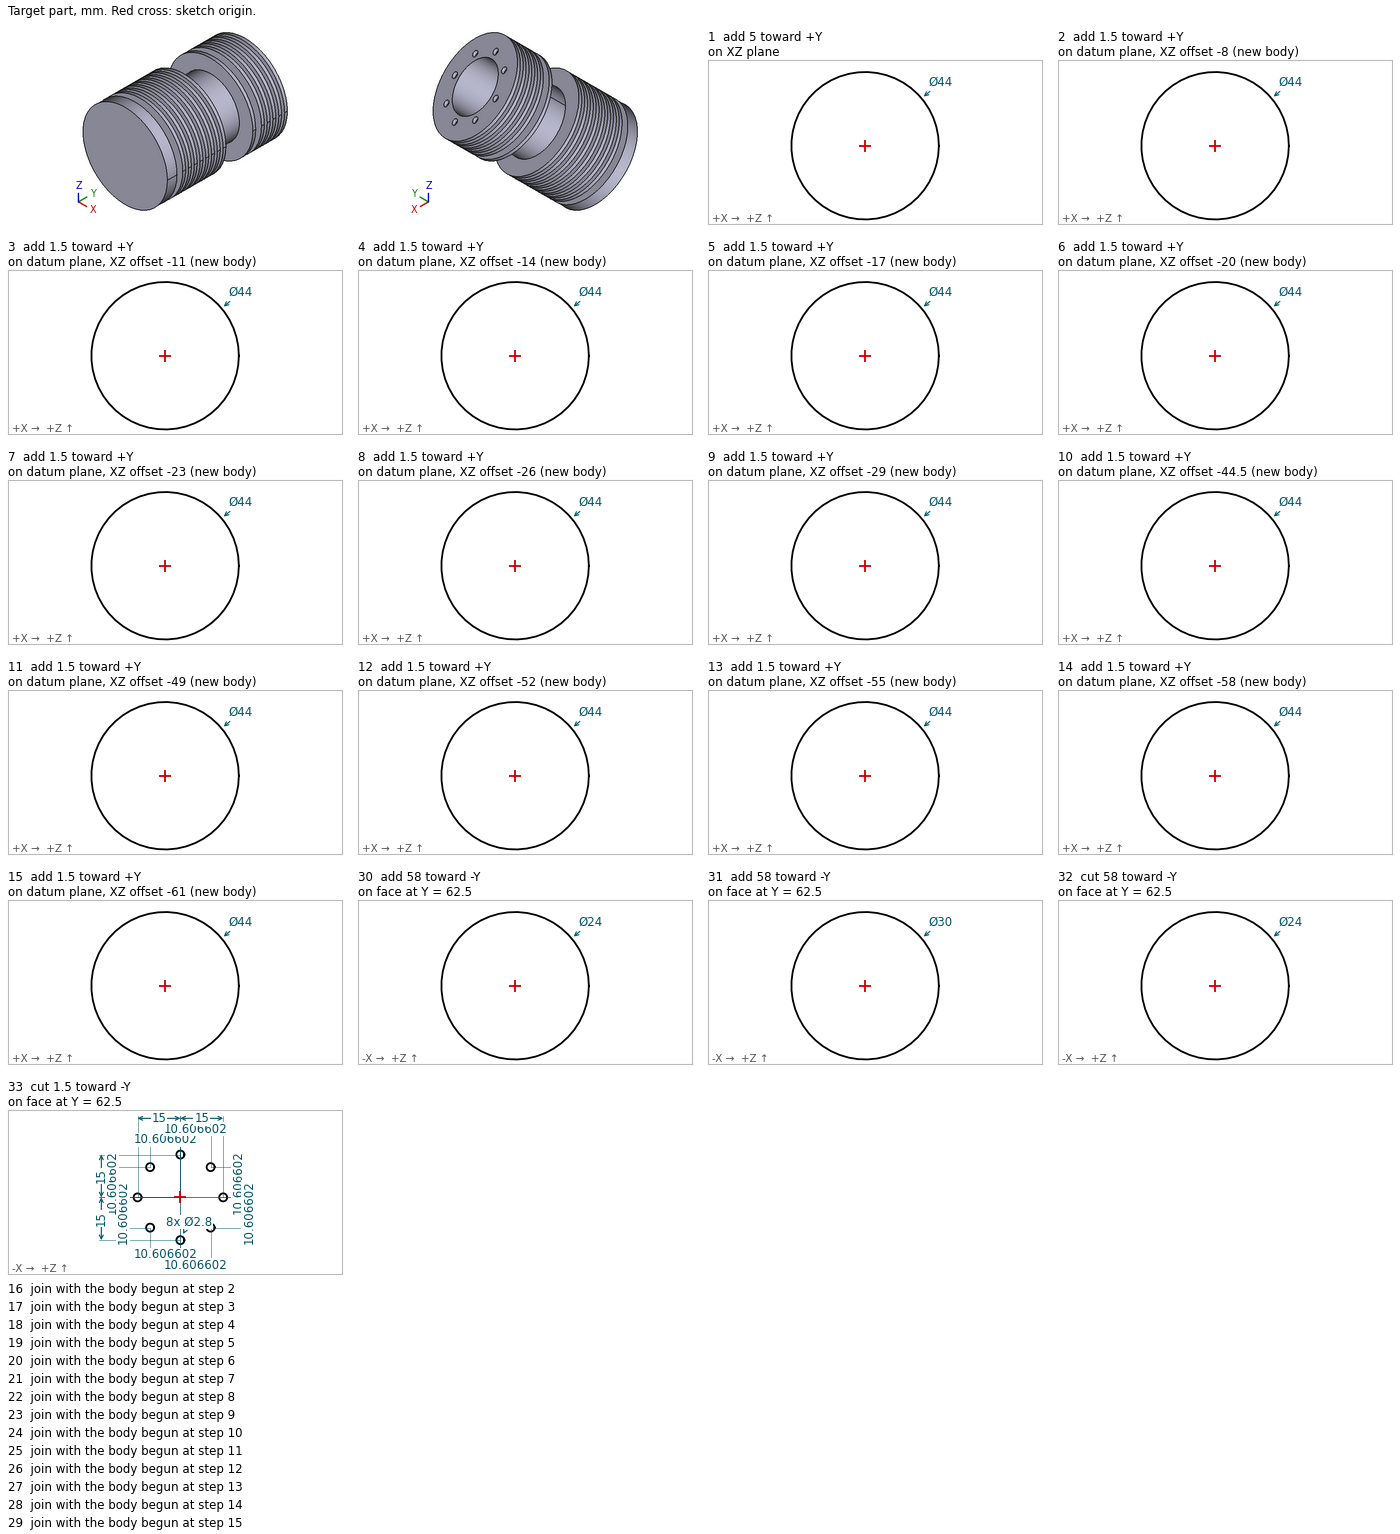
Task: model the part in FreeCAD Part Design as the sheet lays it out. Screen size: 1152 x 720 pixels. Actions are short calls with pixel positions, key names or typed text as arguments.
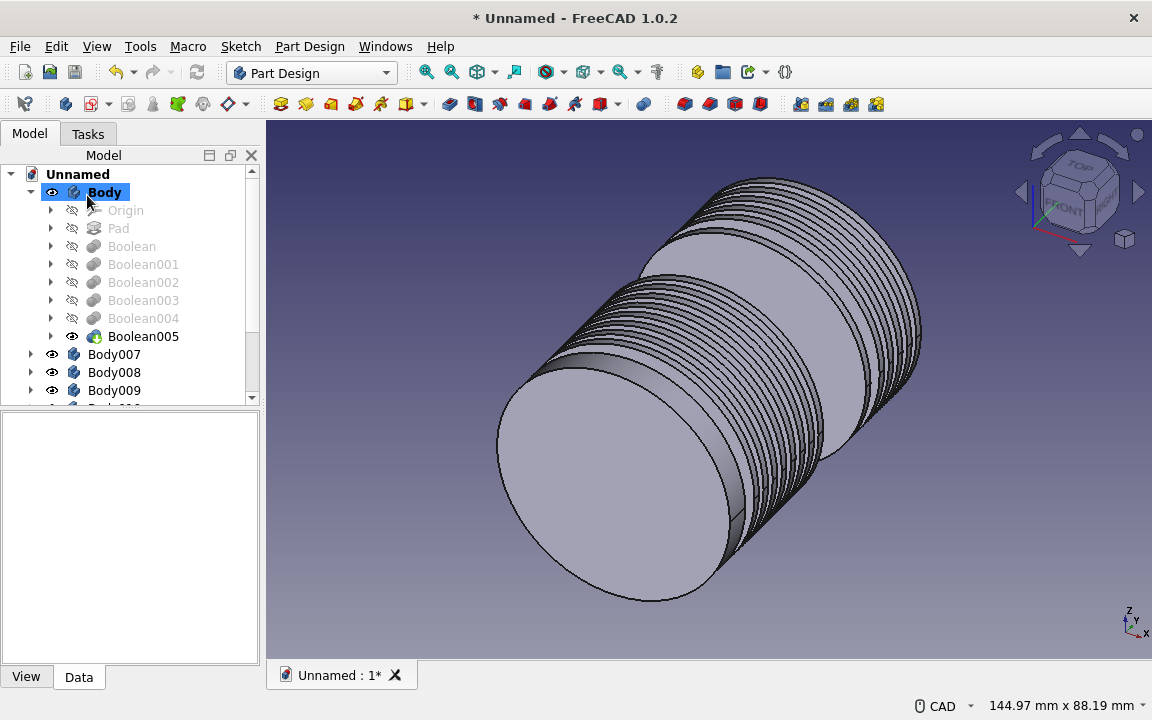
click(97, 354)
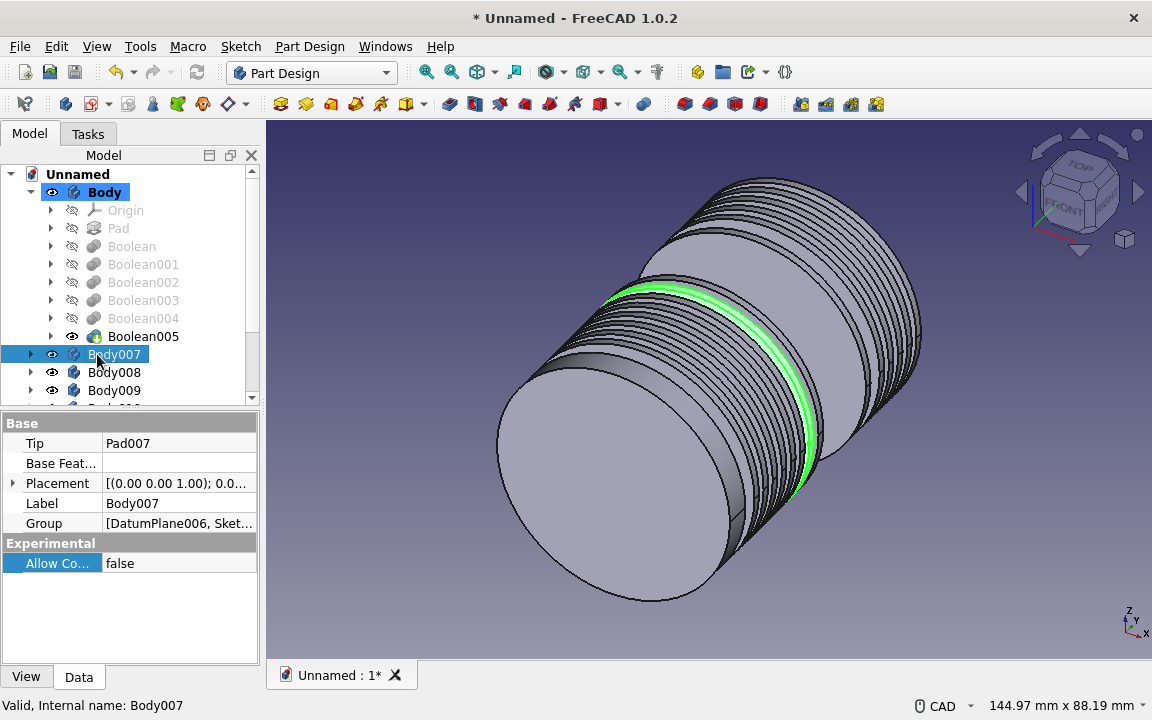
click(644, 104)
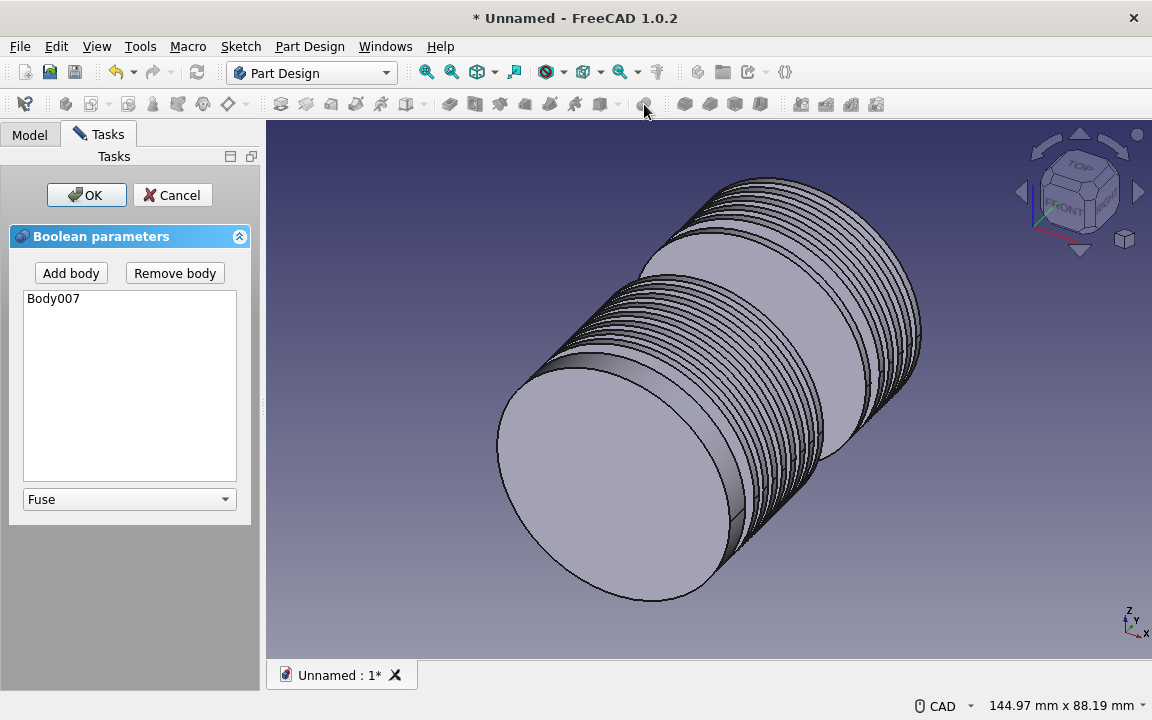
click(87, 195)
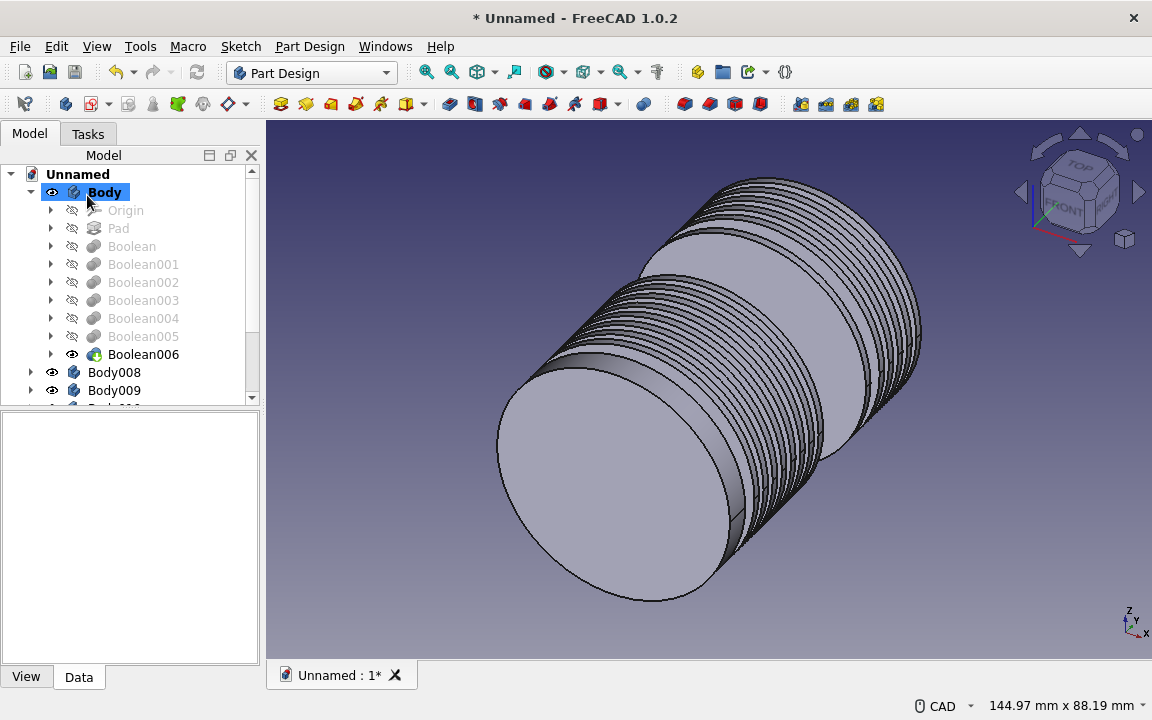
click(97, 372)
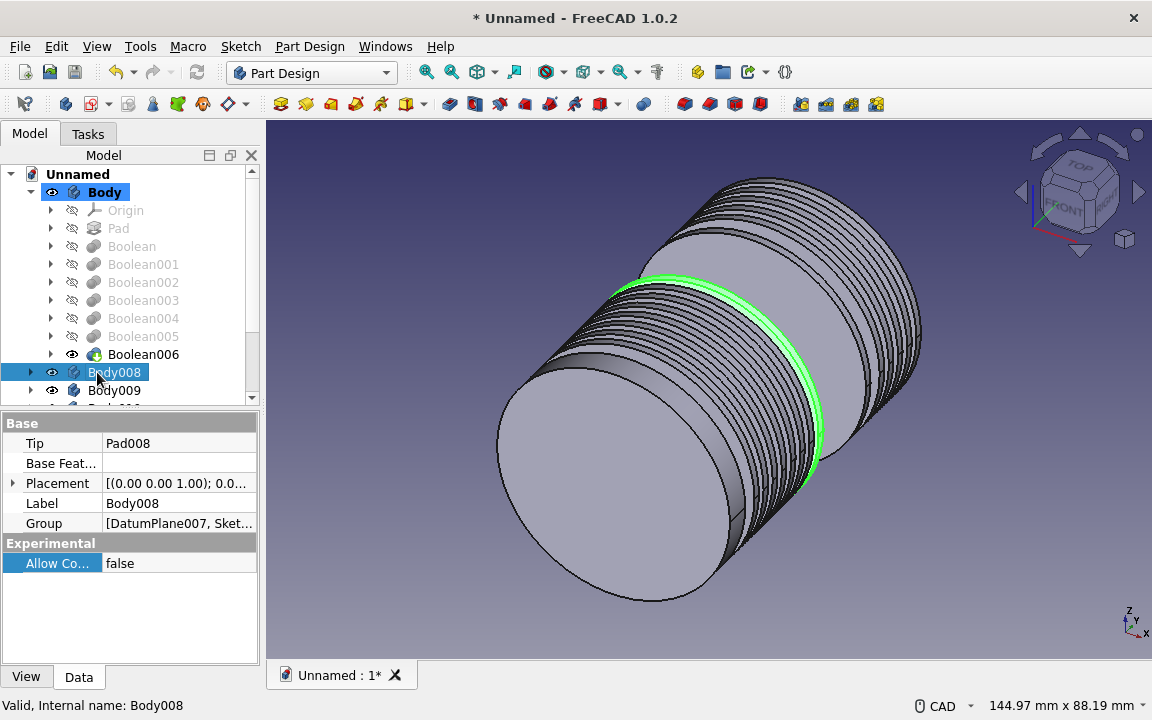
click(644, 104)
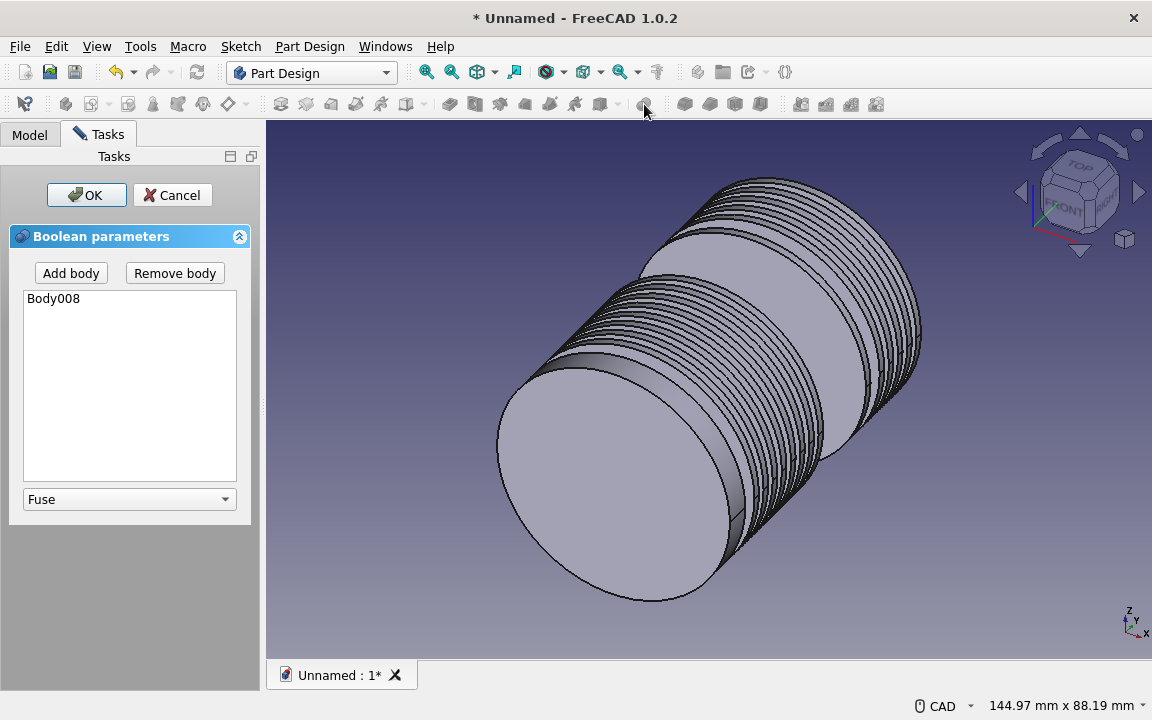
click(87, 195)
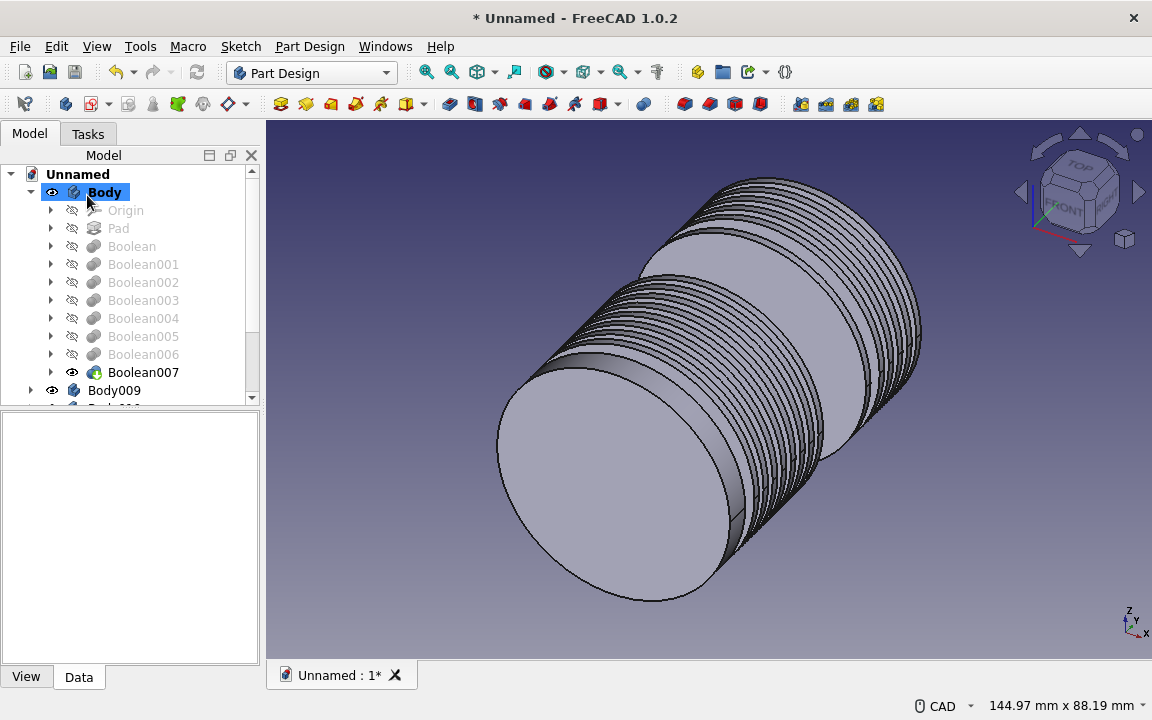
click(97, 390)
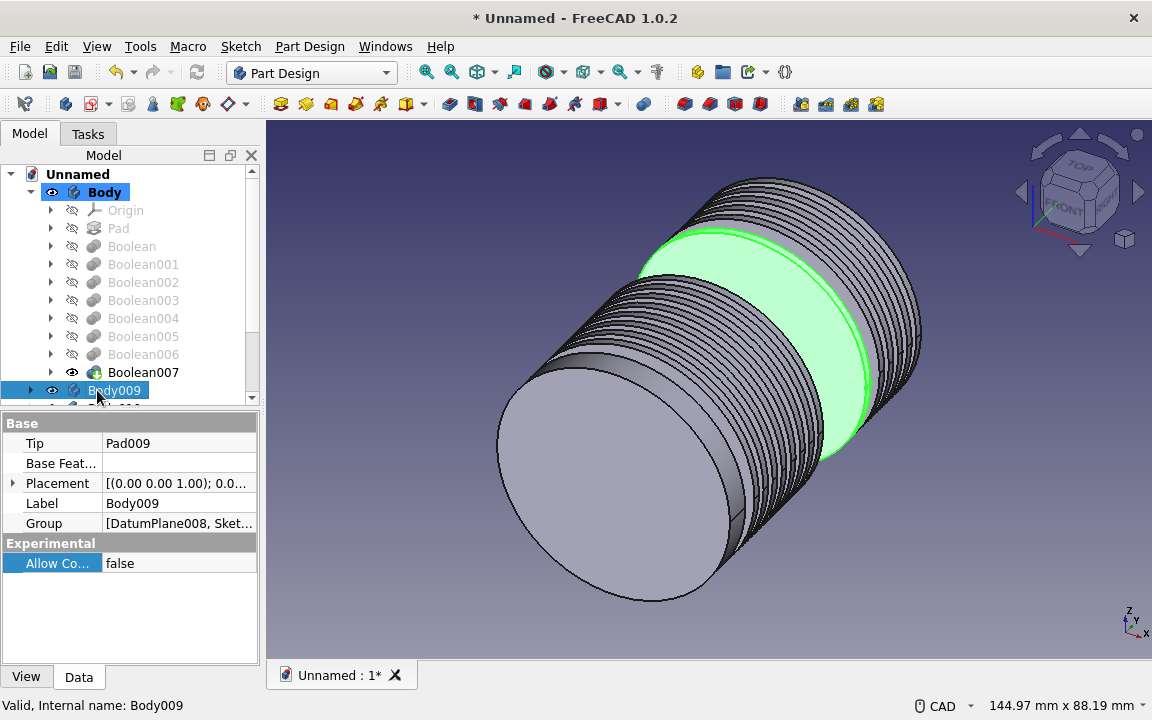
click(644, 104)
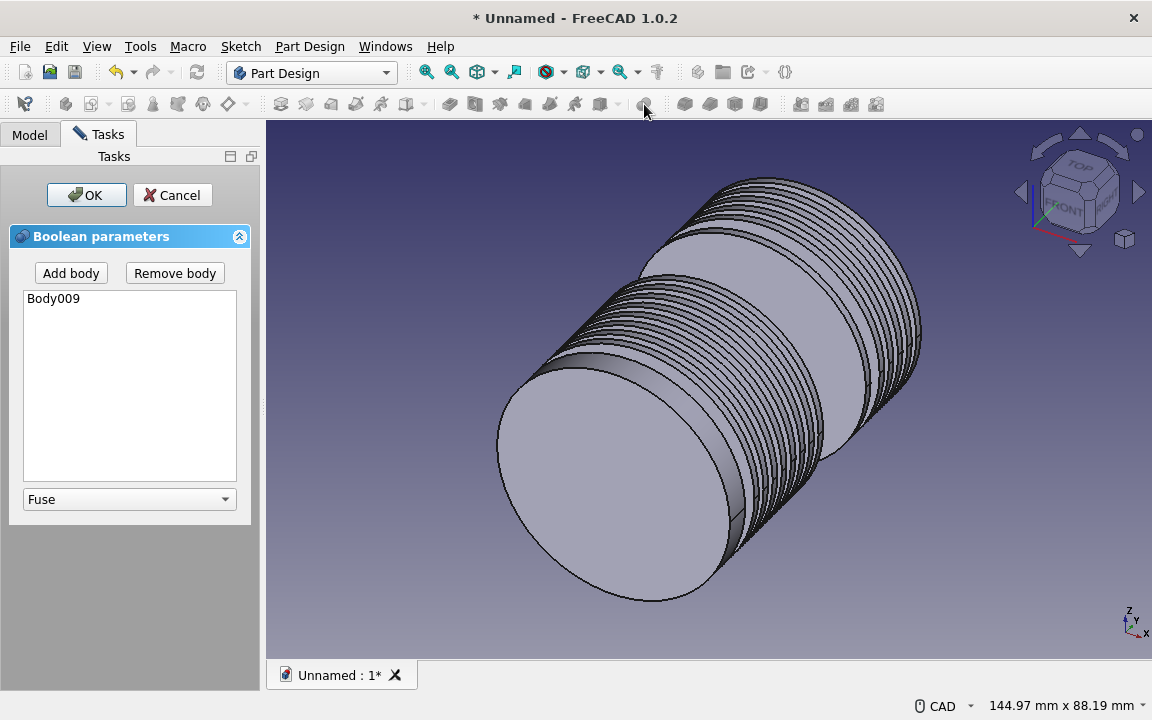
click(87, 195)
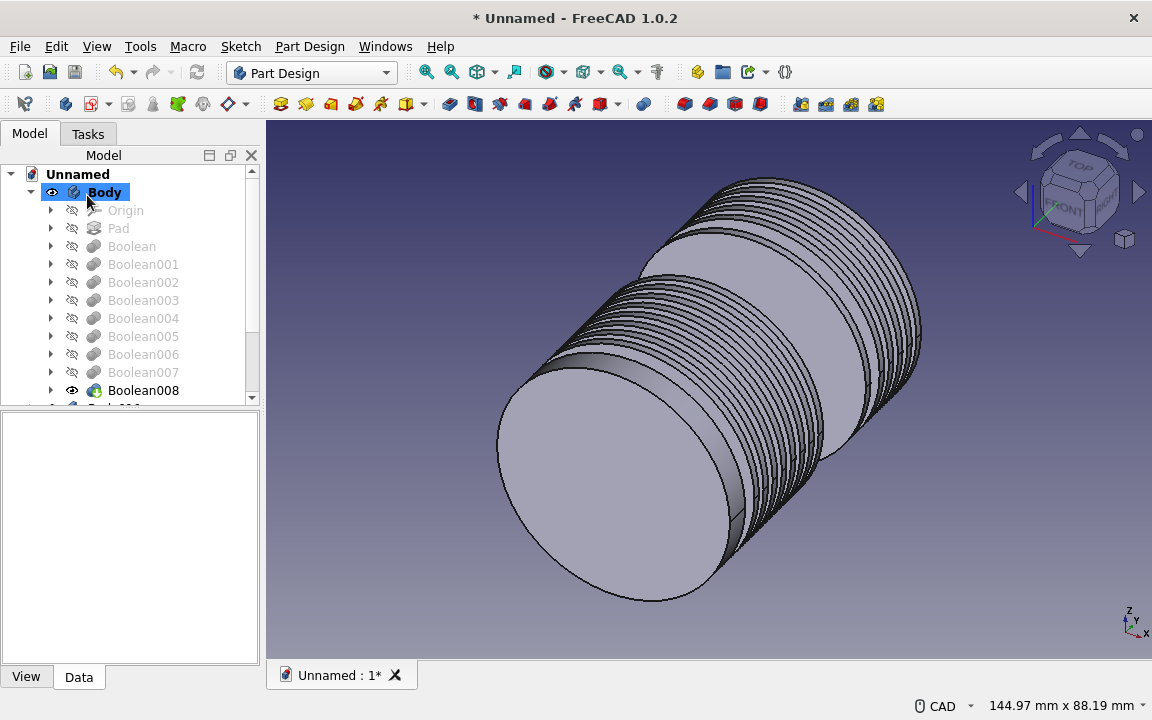
scroll(101, 278, down, 3)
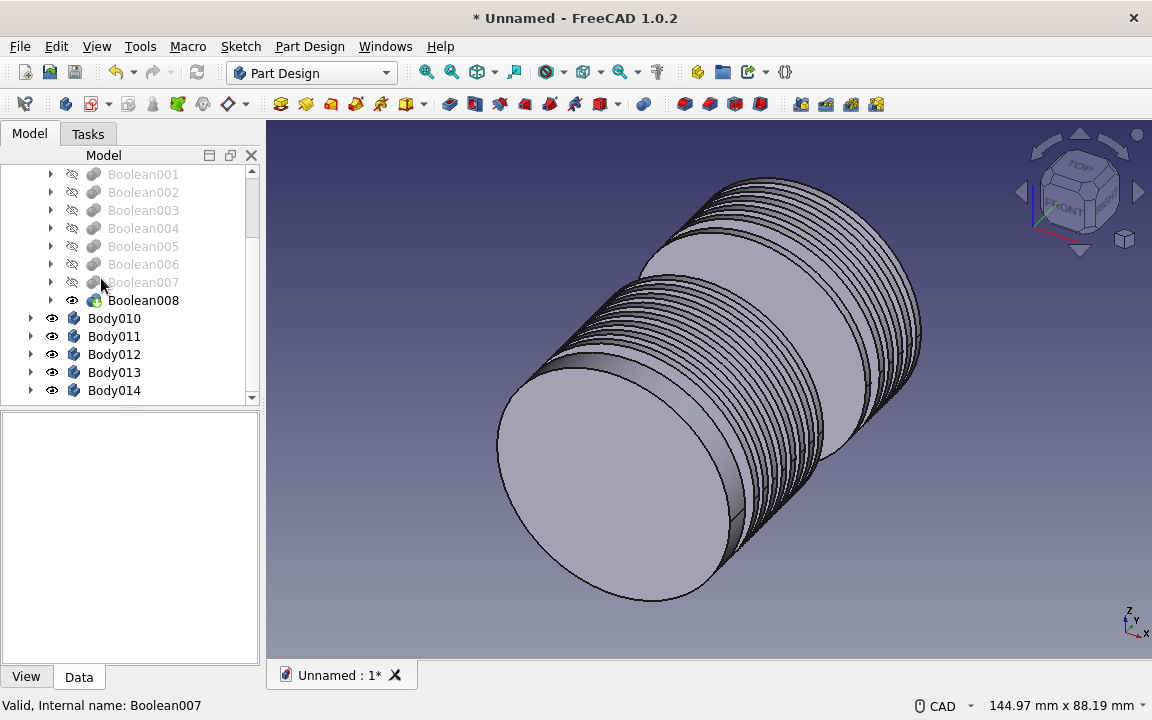
click(97, 318)